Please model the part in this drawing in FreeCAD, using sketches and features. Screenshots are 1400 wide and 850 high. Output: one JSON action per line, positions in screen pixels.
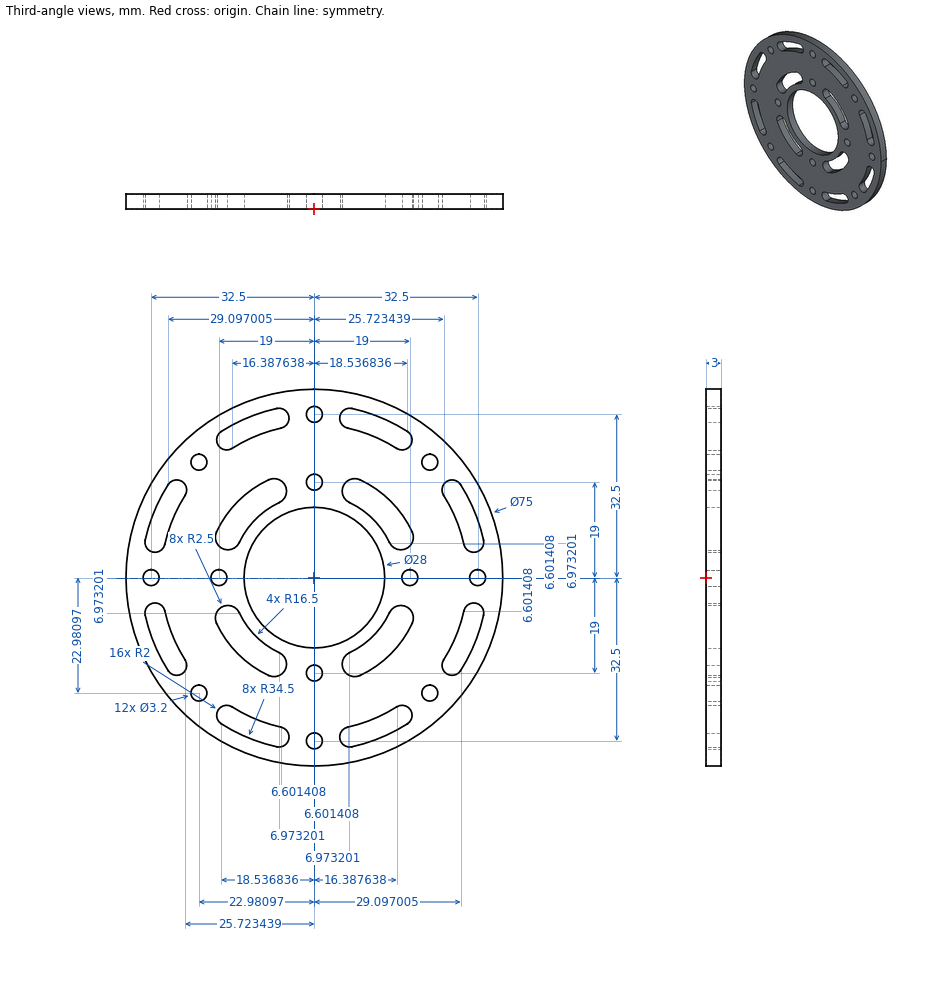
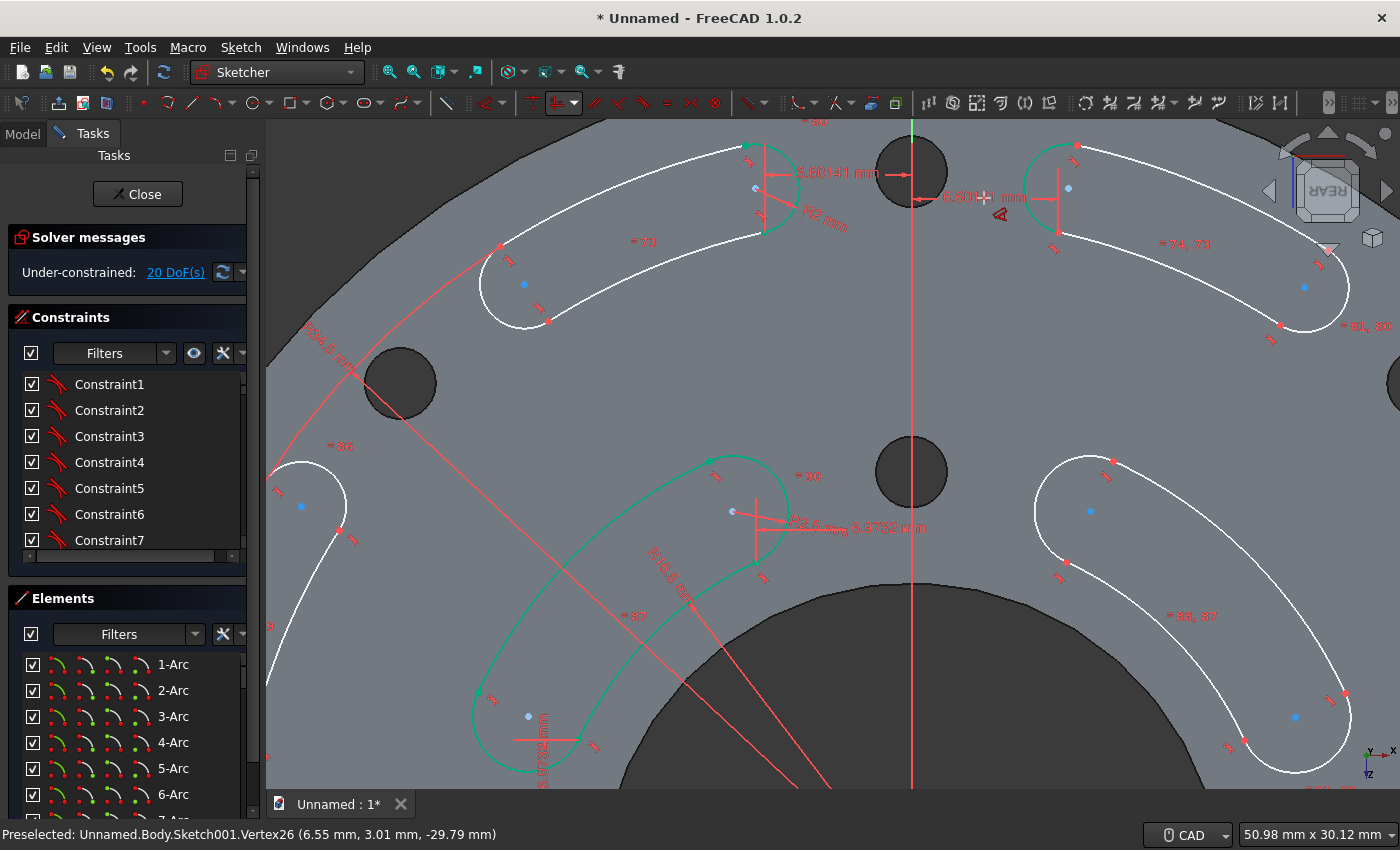
{"action": "scroll", "coordinate": [701, 264], "scroll_direction": "down", "scroll_amount": 6}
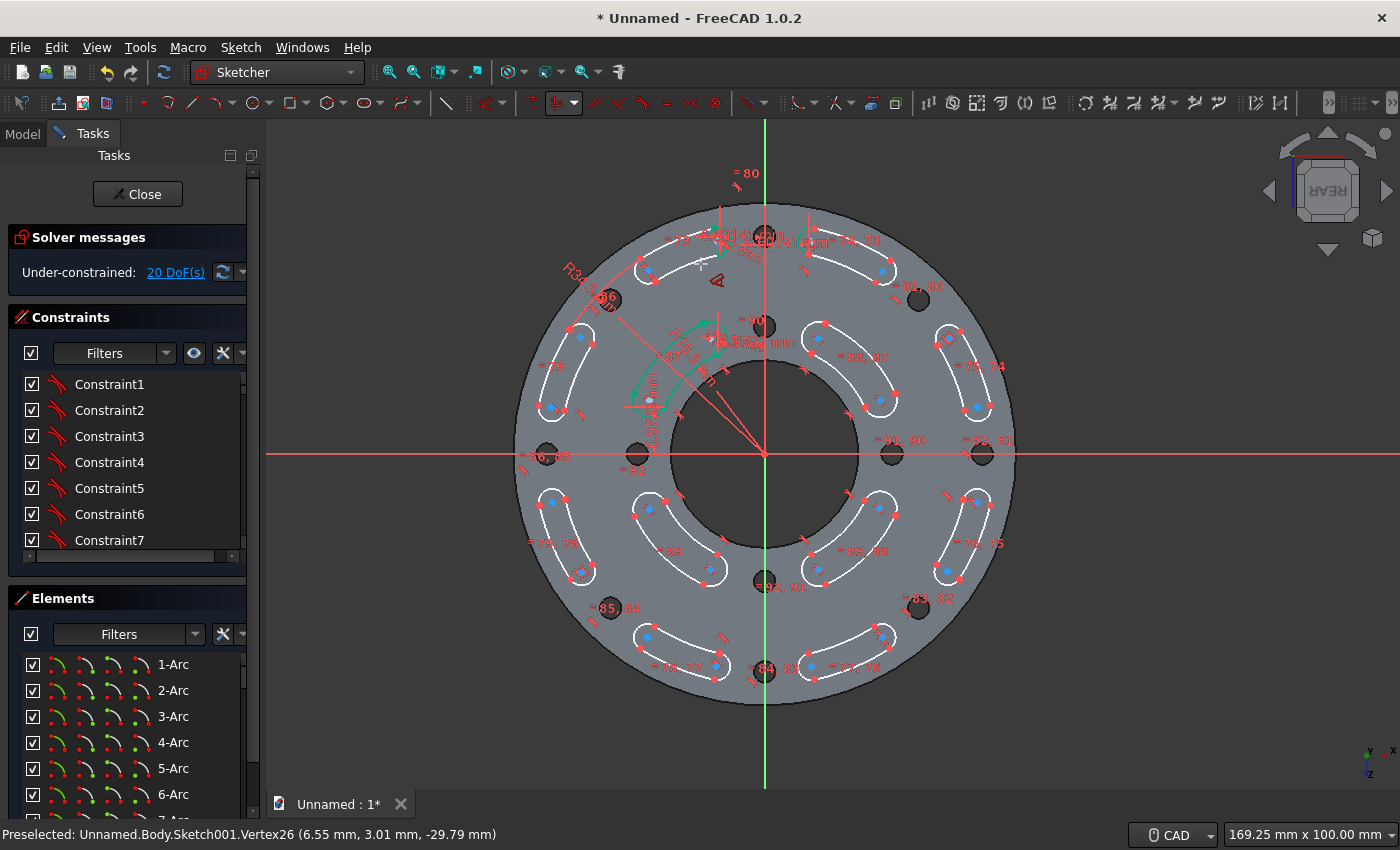
{"action": "left_click", "coordinate": [964, 411]}
{"action": "left_click", "coordinate": [998, 432]}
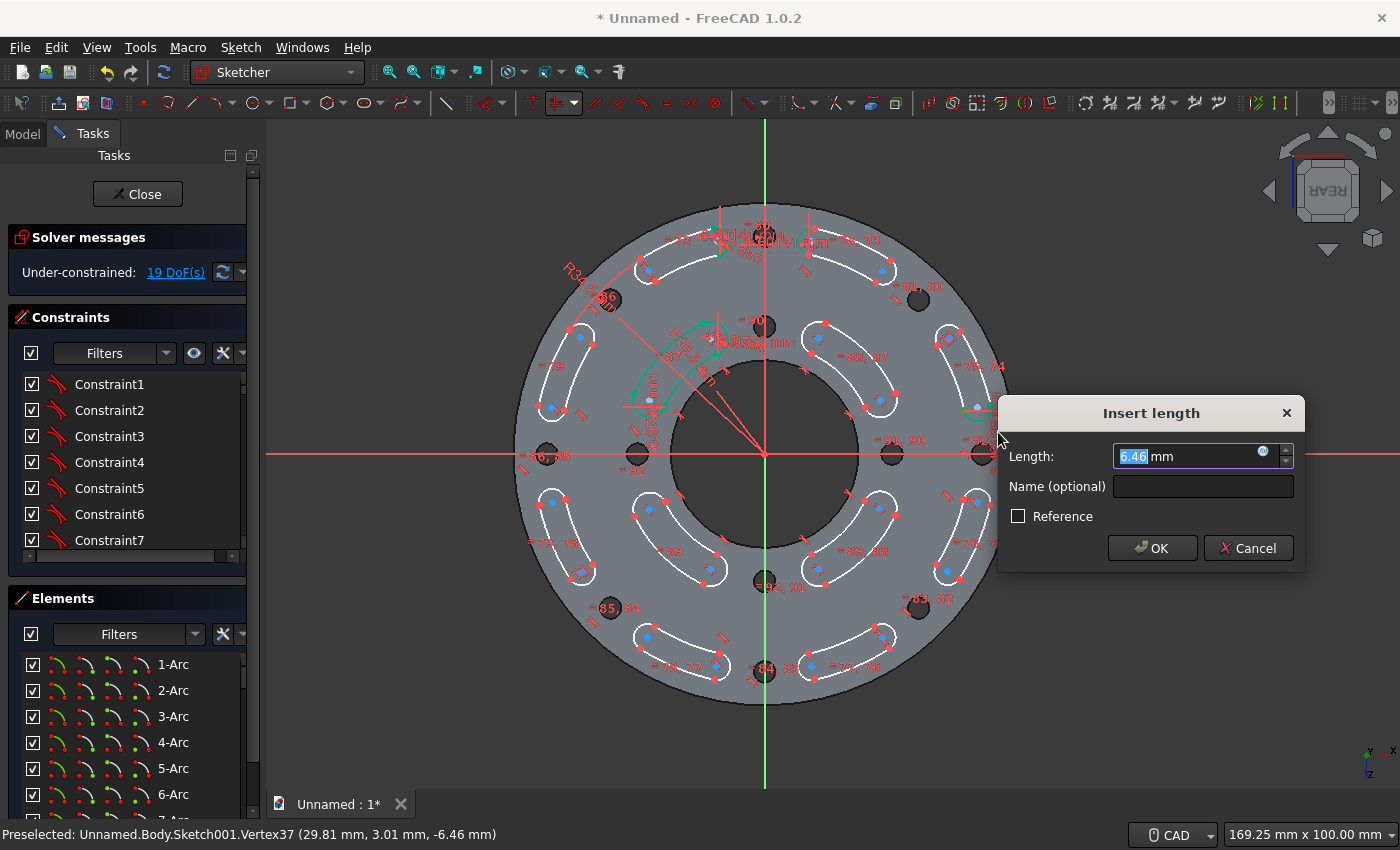
{"action": "type", "text": "6.601408"}
{"action": "key", "text": "Return"}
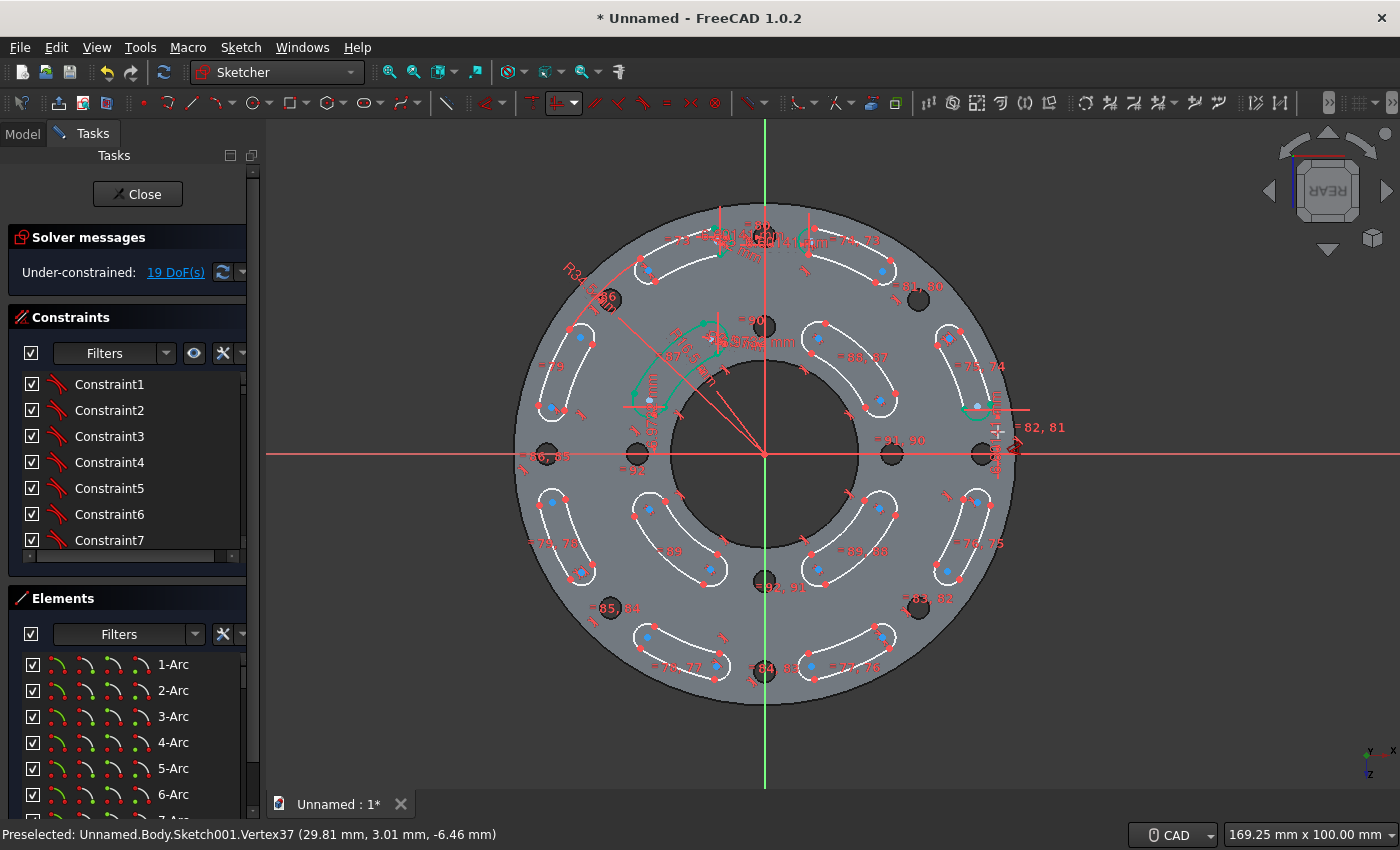
{"action": "left_click", "coordinate": [964, 499]}
{"action": "left_click", "coordinate": [998, 477]}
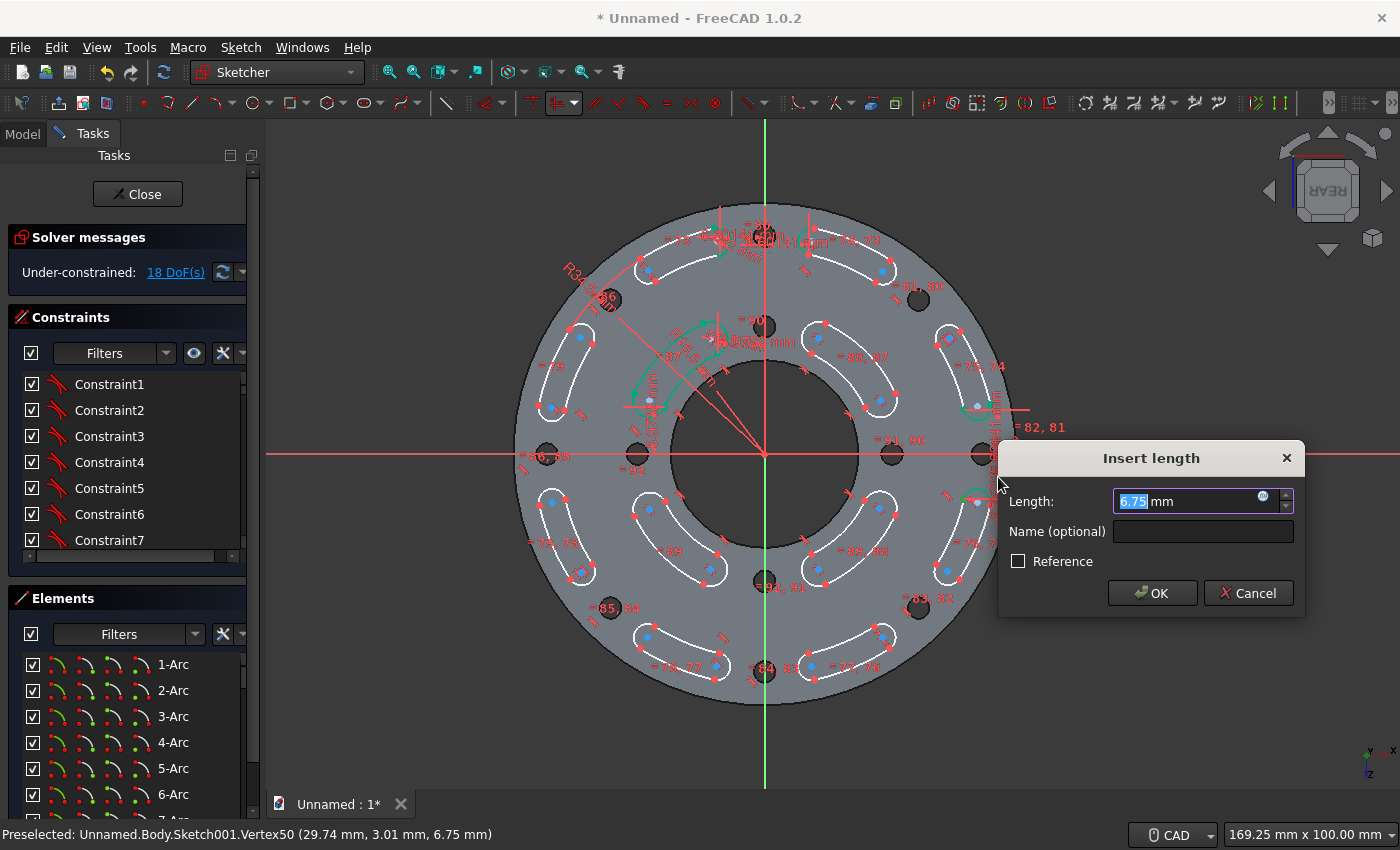
{"action": "type", "text": "6.601408"}
{"action": "key", "text": "Return"}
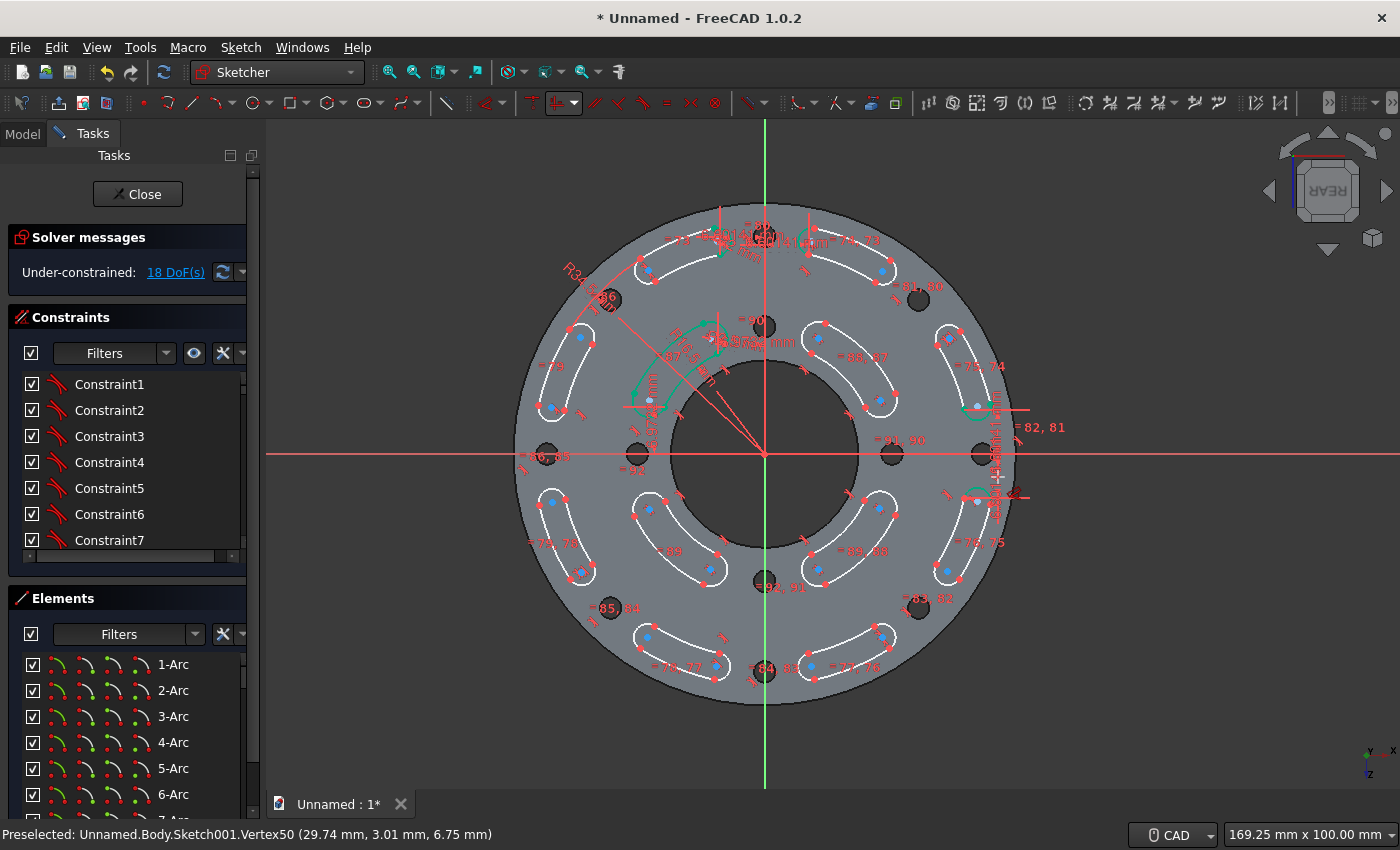
{"action": "left_click", "coordinate": [809, 654]}
{"action": "left_click", "coordinate": [787, 688]}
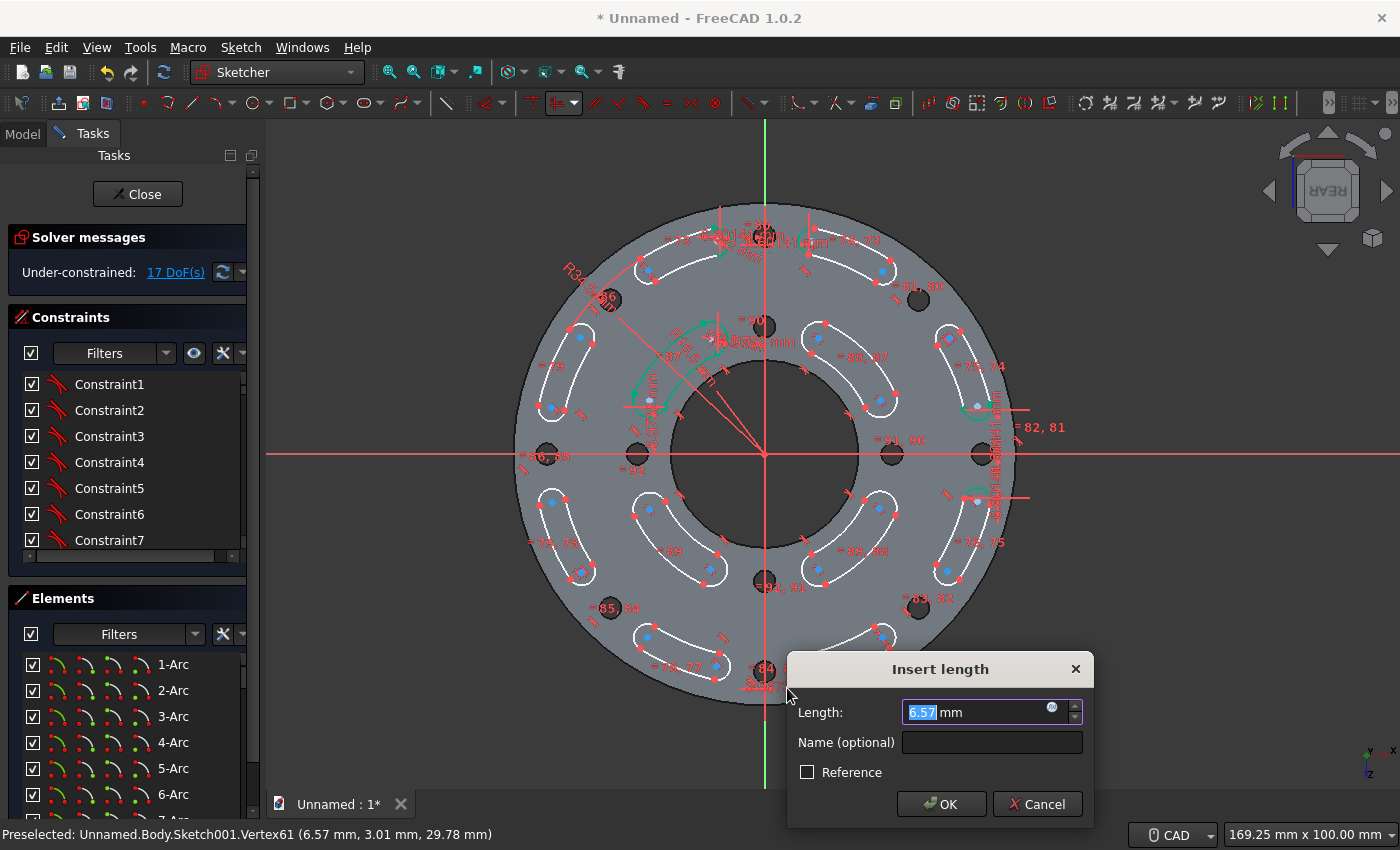
{"action": "type", "text": "6.601408"}
{"action": "key", "text": "Return"}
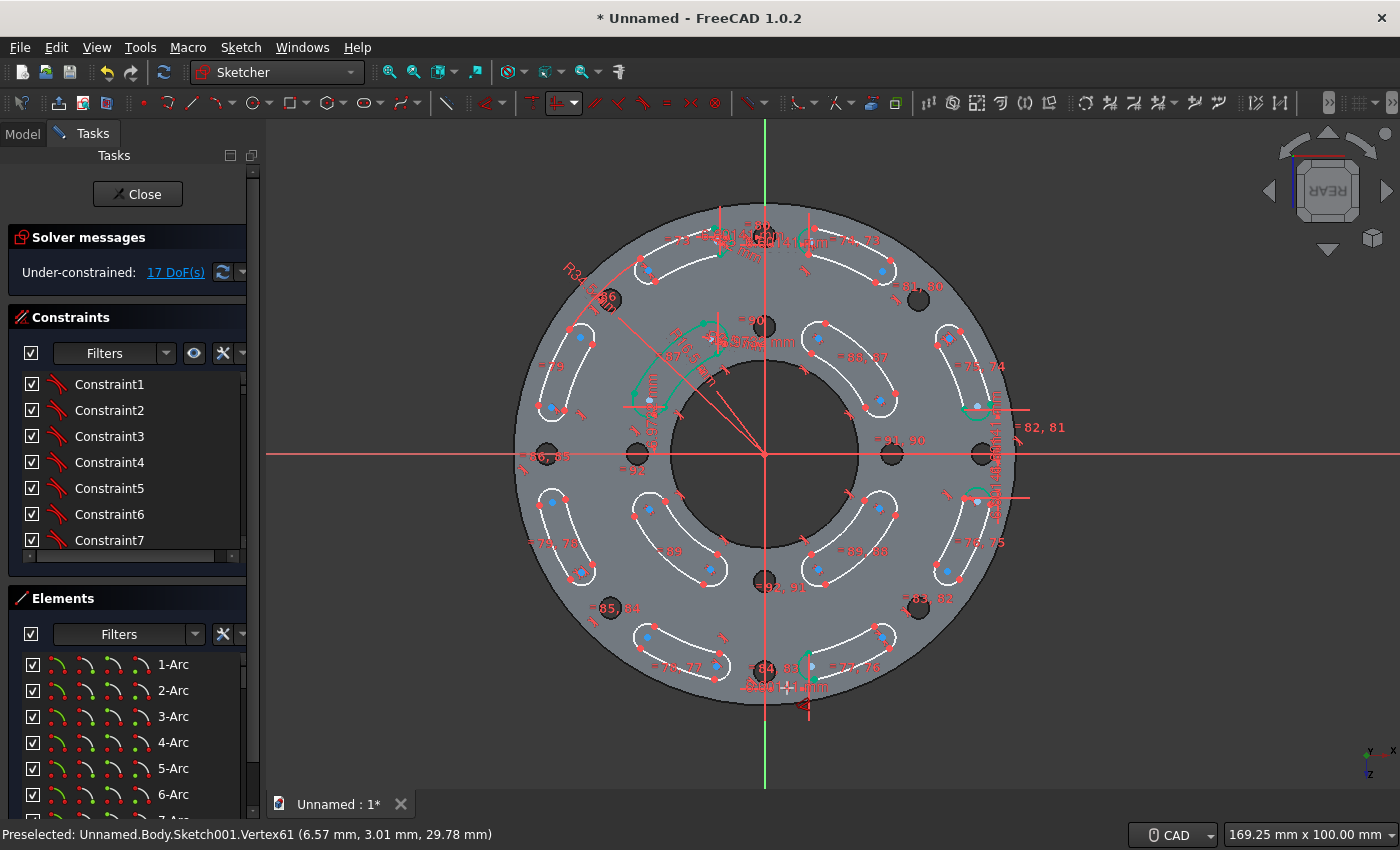
{"action": "left_click", "coordinate": [720, 653]}
{"action": "left_click", "coordinate": [742, 420]}